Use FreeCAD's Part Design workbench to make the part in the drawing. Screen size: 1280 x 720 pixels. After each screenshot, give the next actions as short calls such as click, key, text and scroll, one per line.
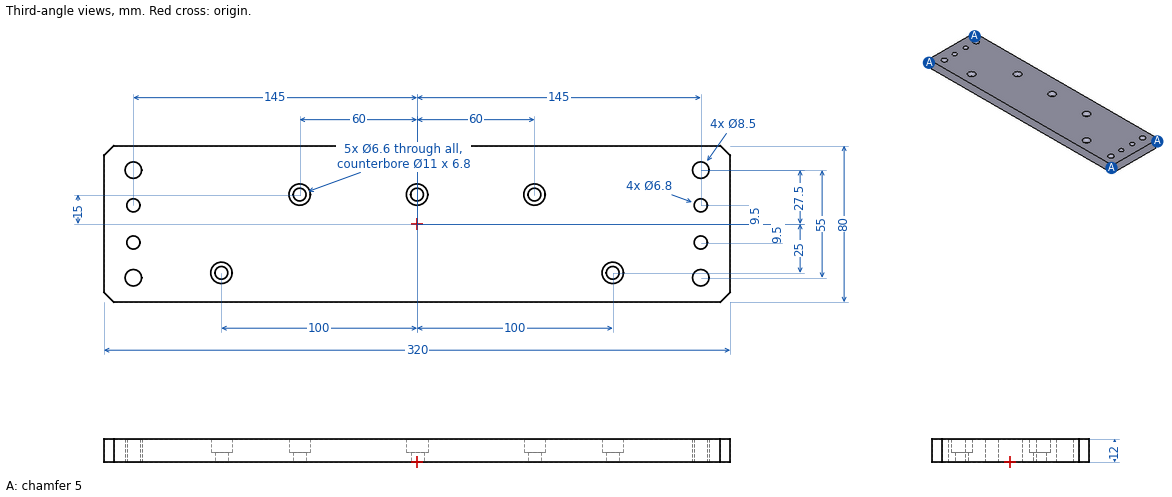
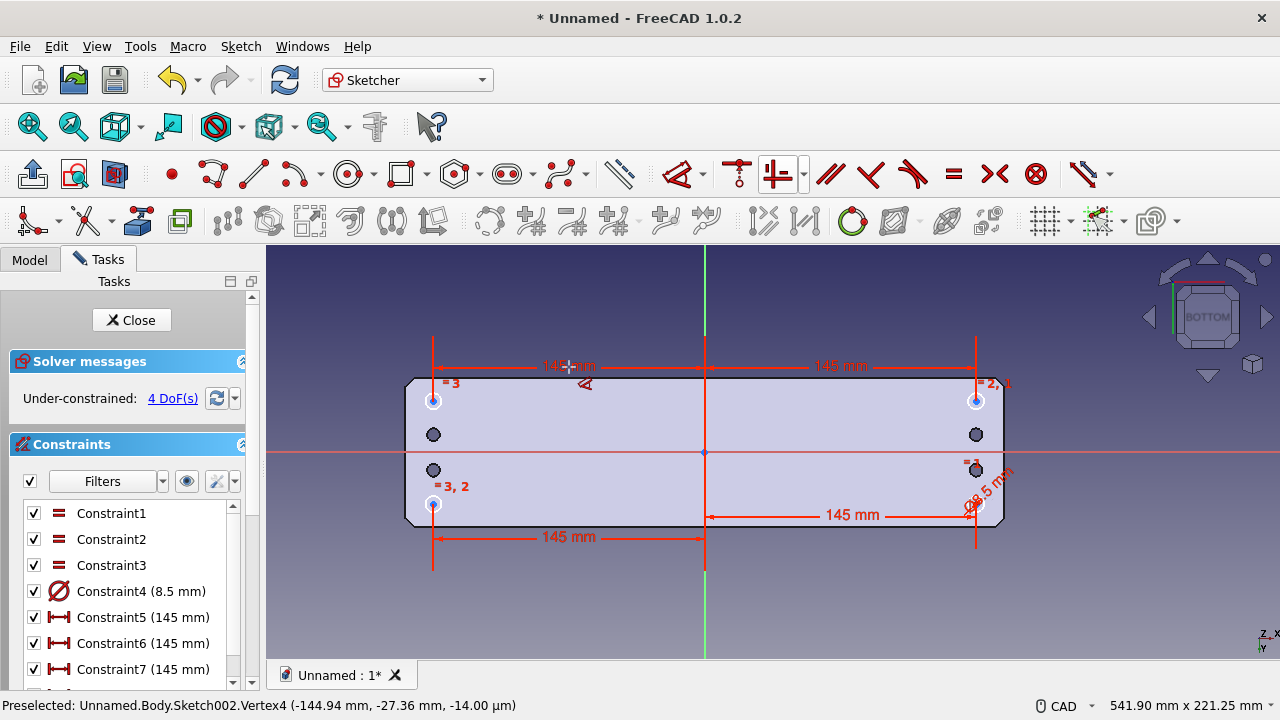
click(976, 504)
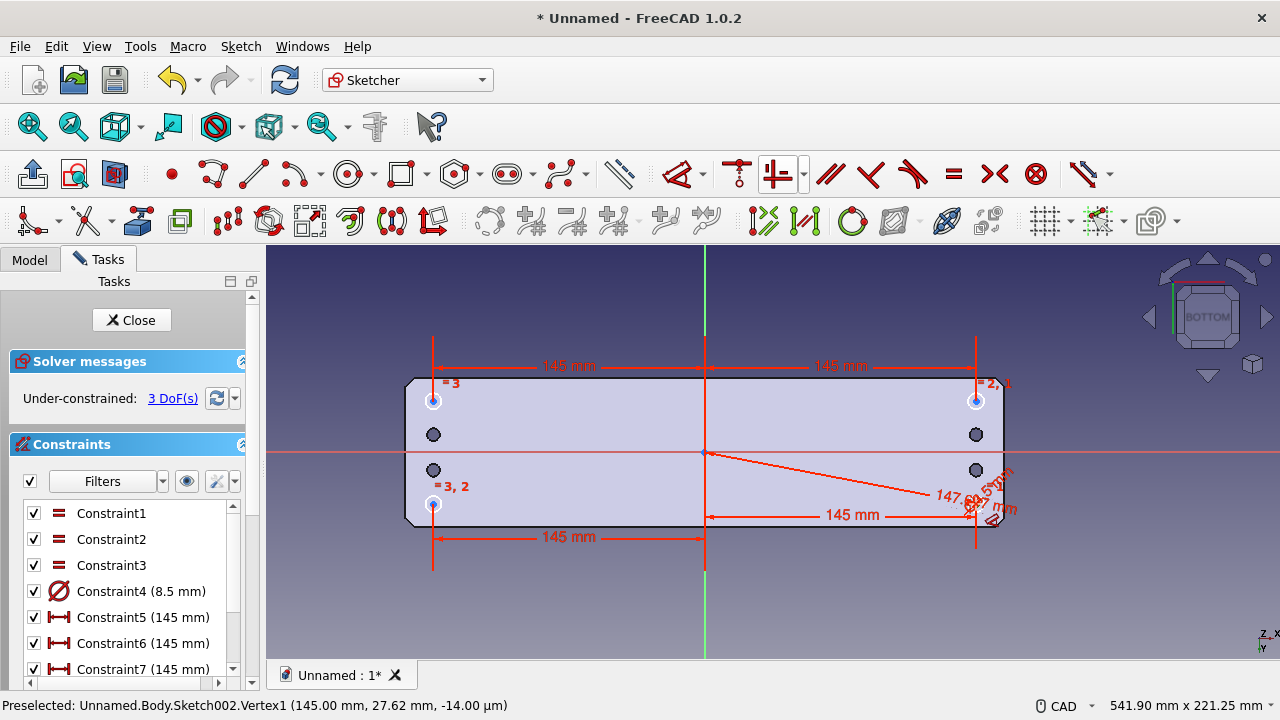
click(976, 401)
click(1010, 429)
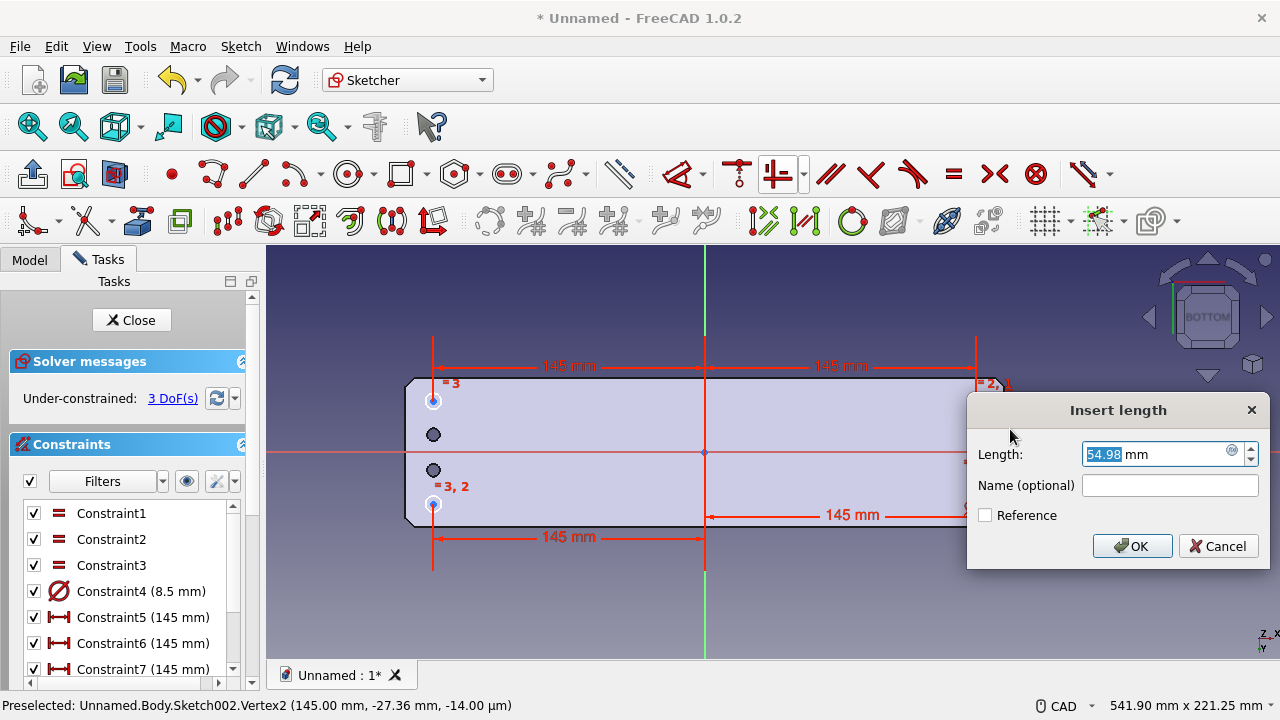
text(55)
key(Return)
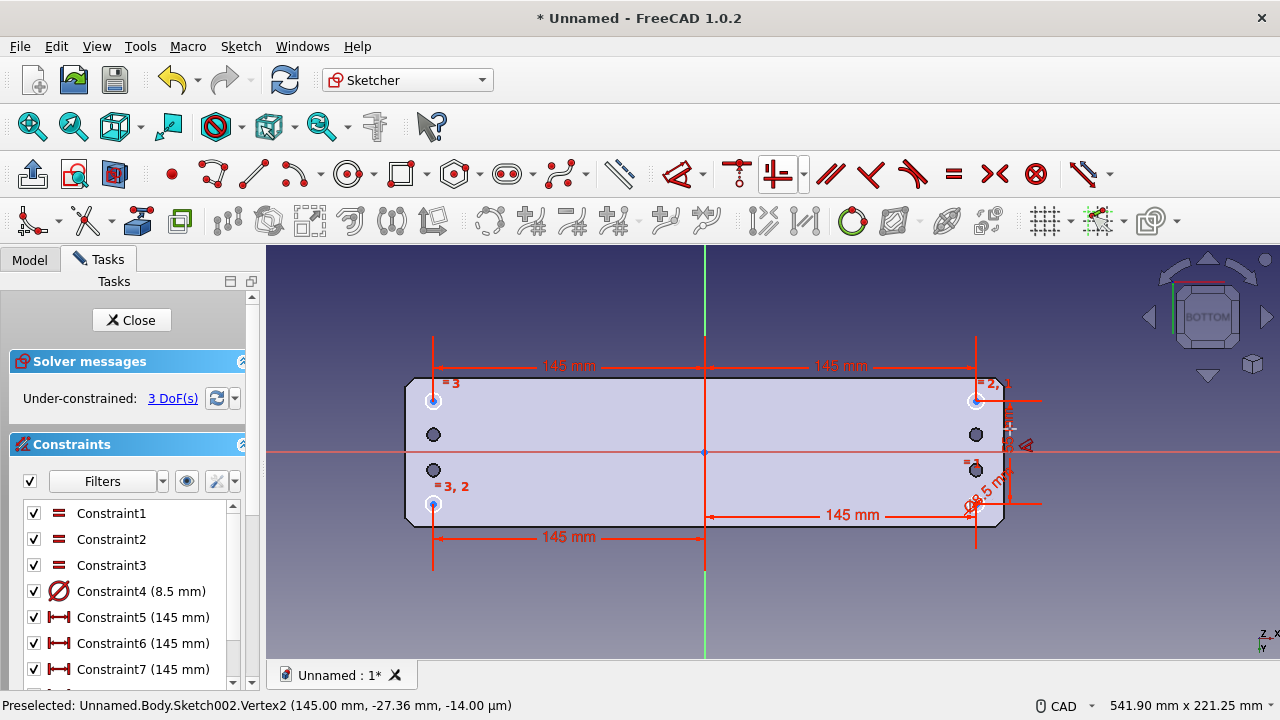
click(976, 401)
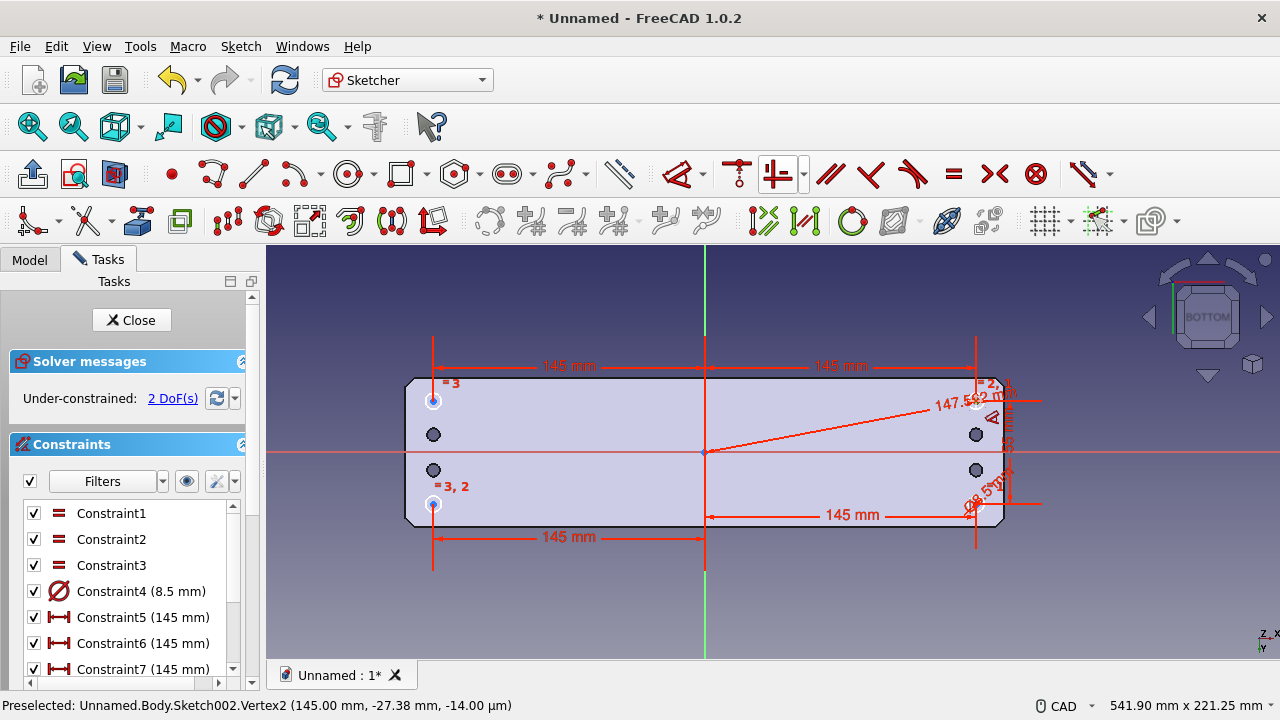
click(433, 504)
click(399, 429)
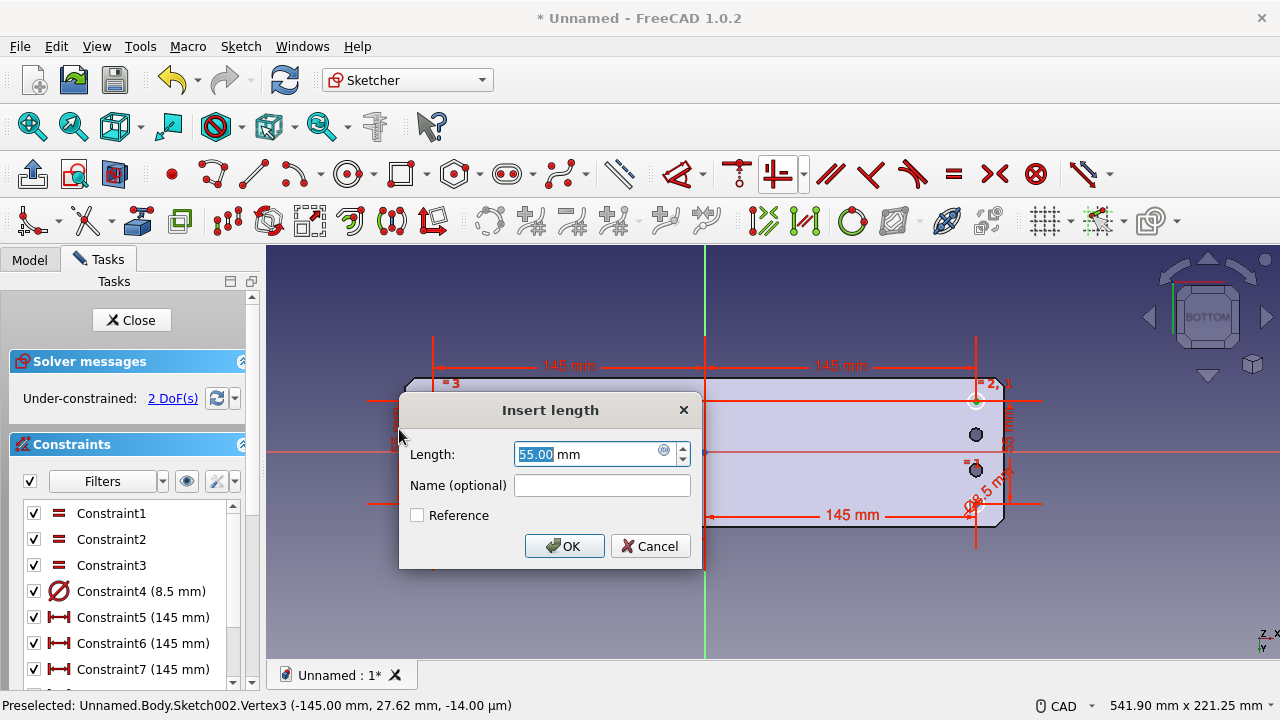
text(55)
key(Return)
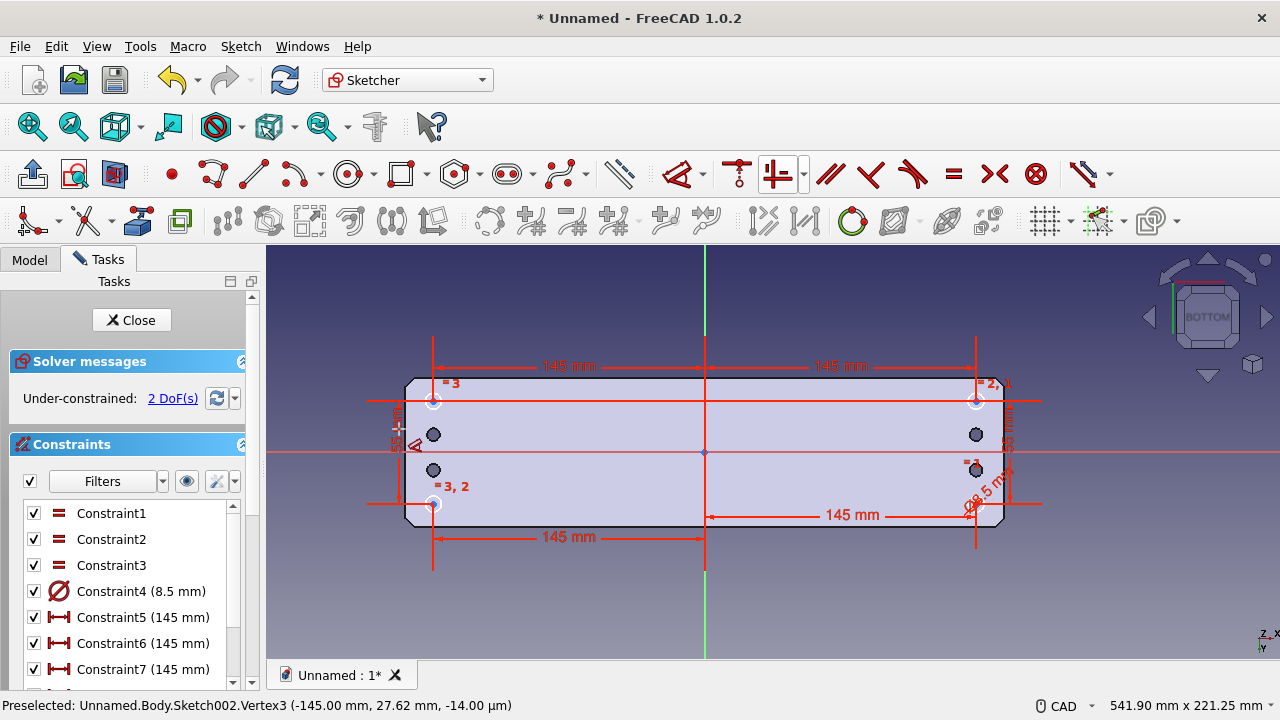
click(433, 504)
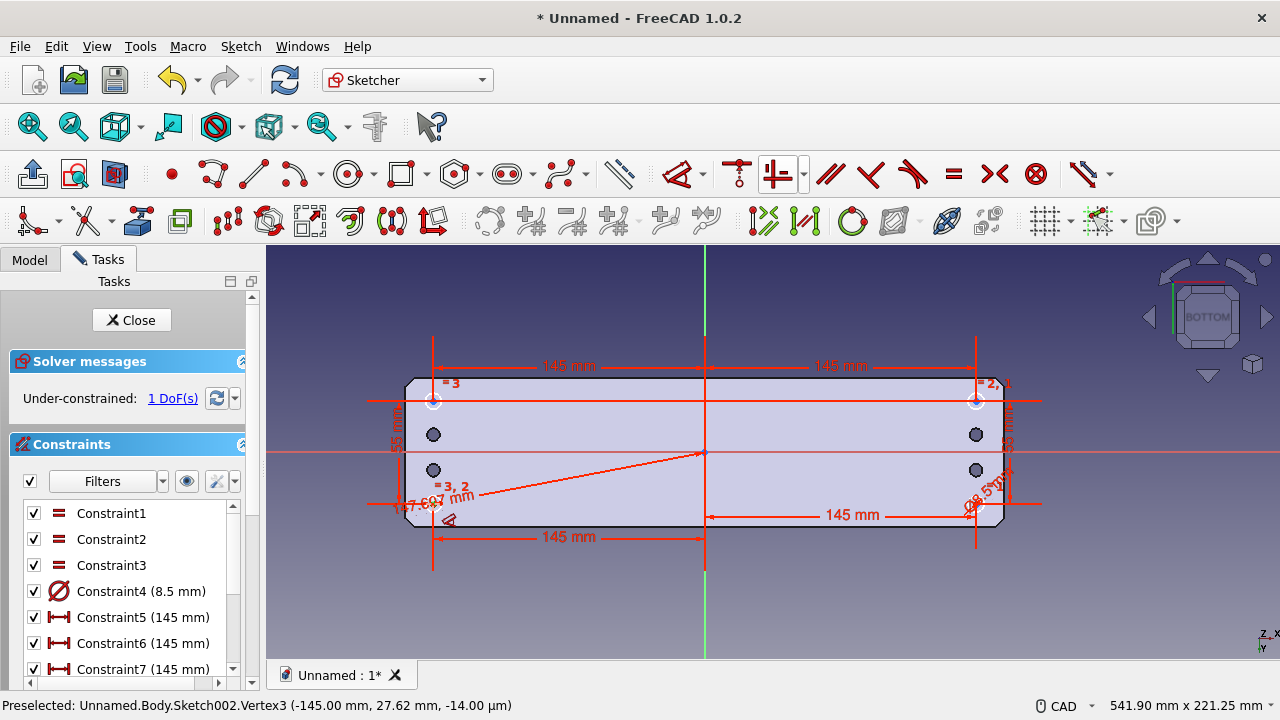
click(433, 401)
click(399, 476)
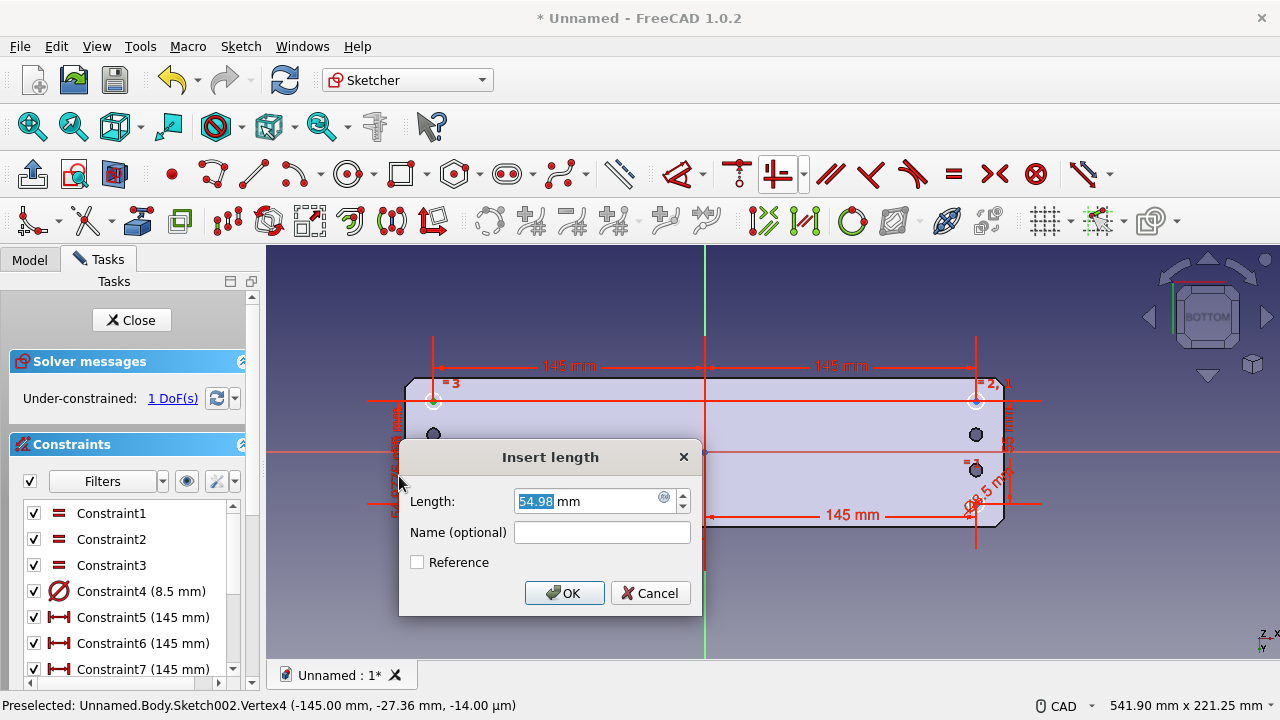
text(55)
key(Return)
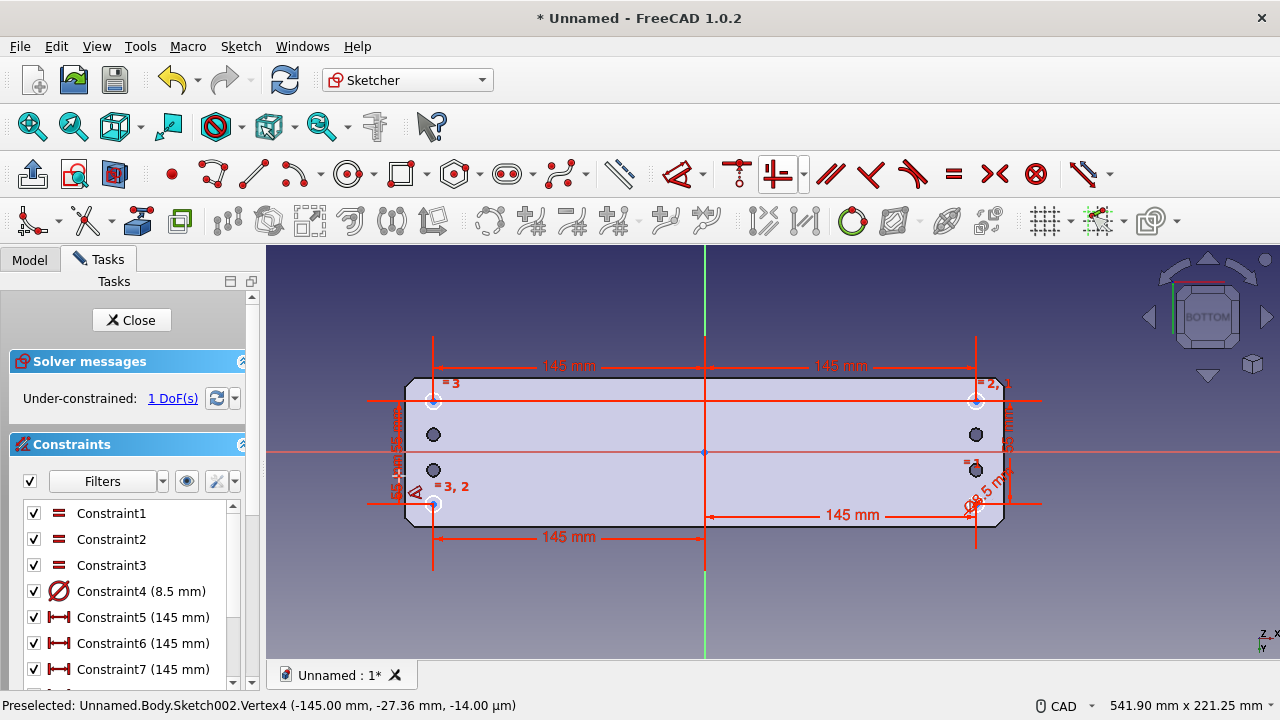
click(976, 504)
click(1010, 466)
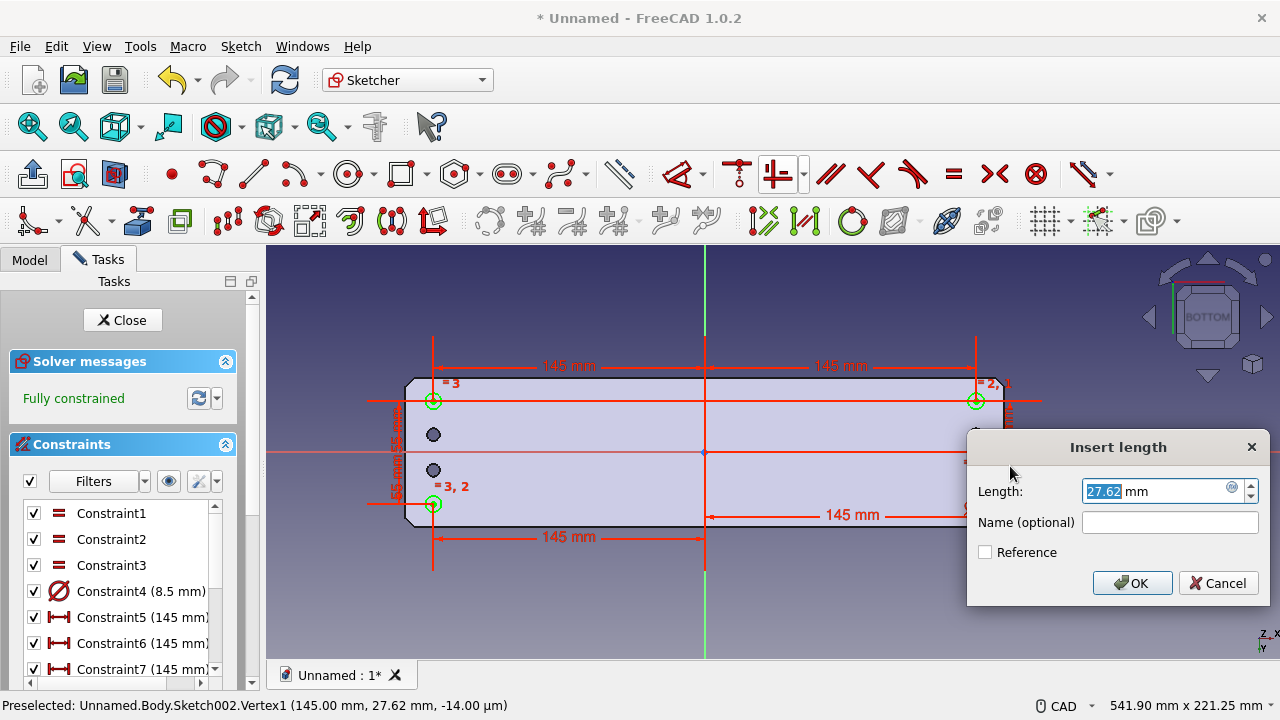
text(27.5)
key(Return)
key(Escape)